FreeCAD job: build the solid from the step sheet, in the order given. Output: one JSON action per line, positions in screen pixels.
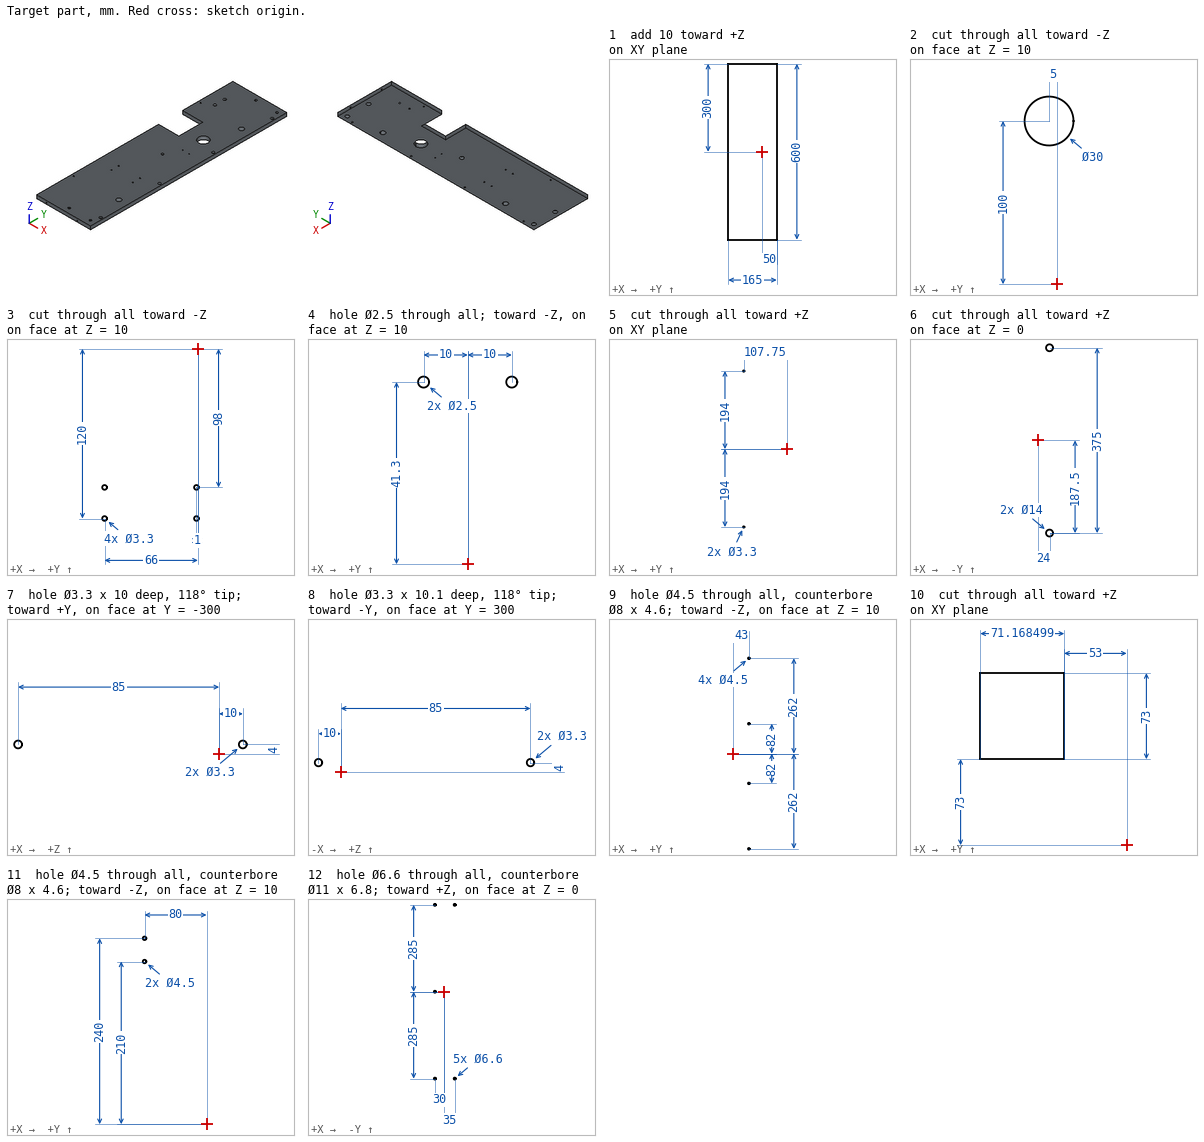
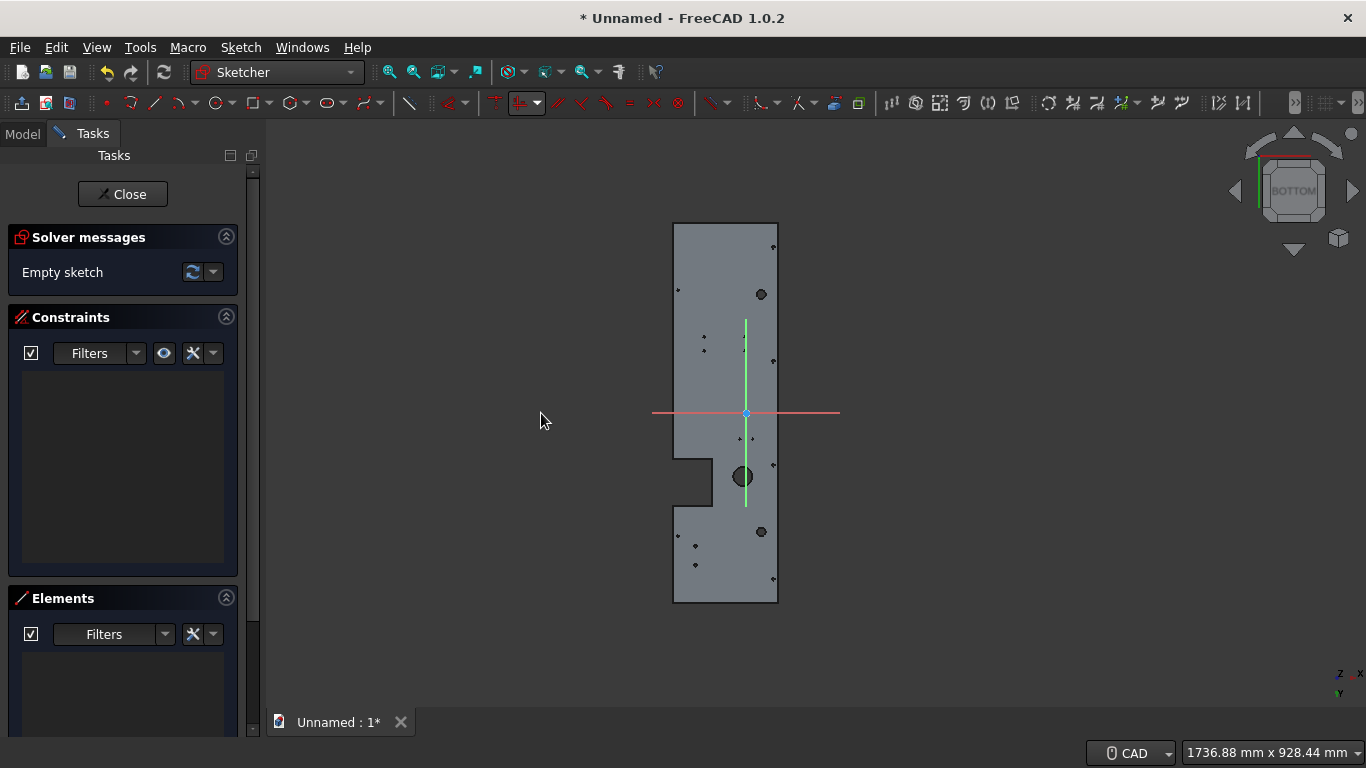
{"action": "left_click", "coordinate": [216, 104]}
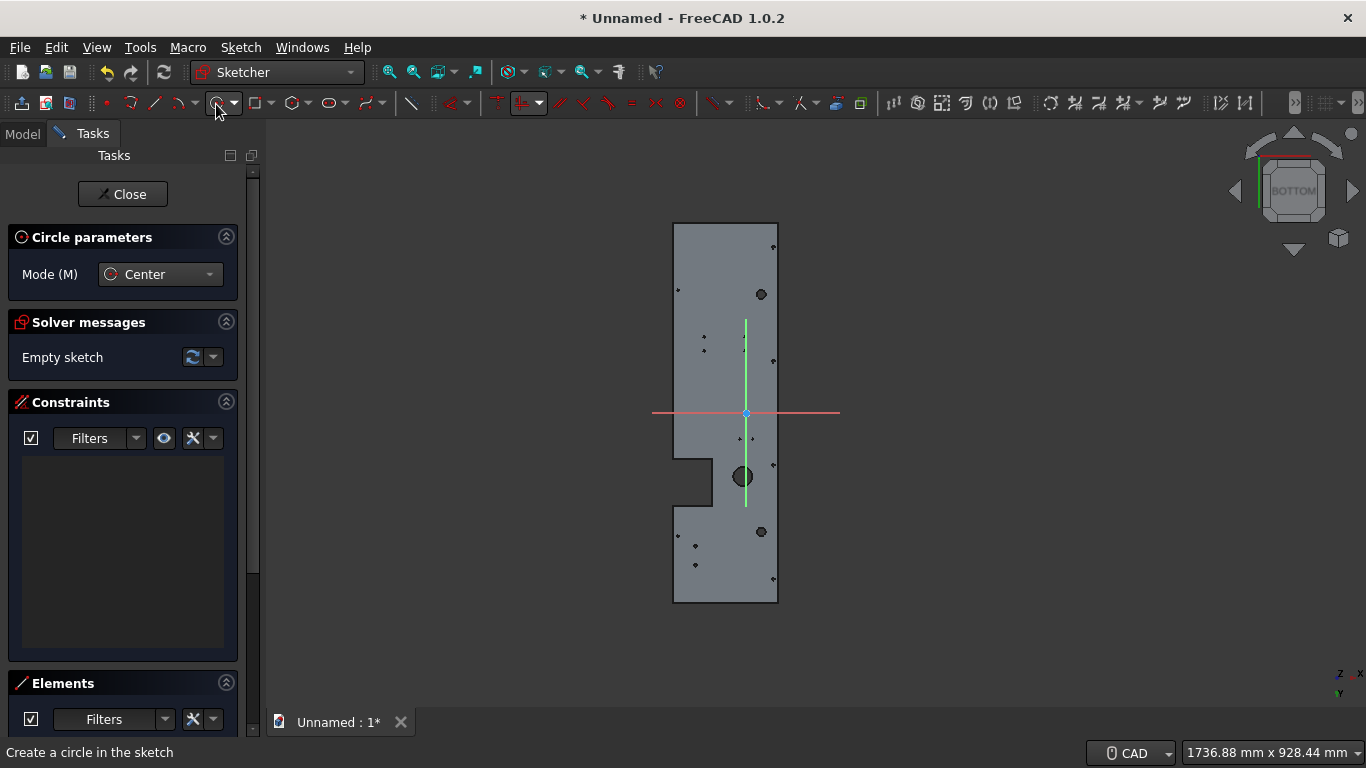
{"action": "scroll", "coordinate": [727, 594], "scroll_direction": "up", "scroll_amount": 12}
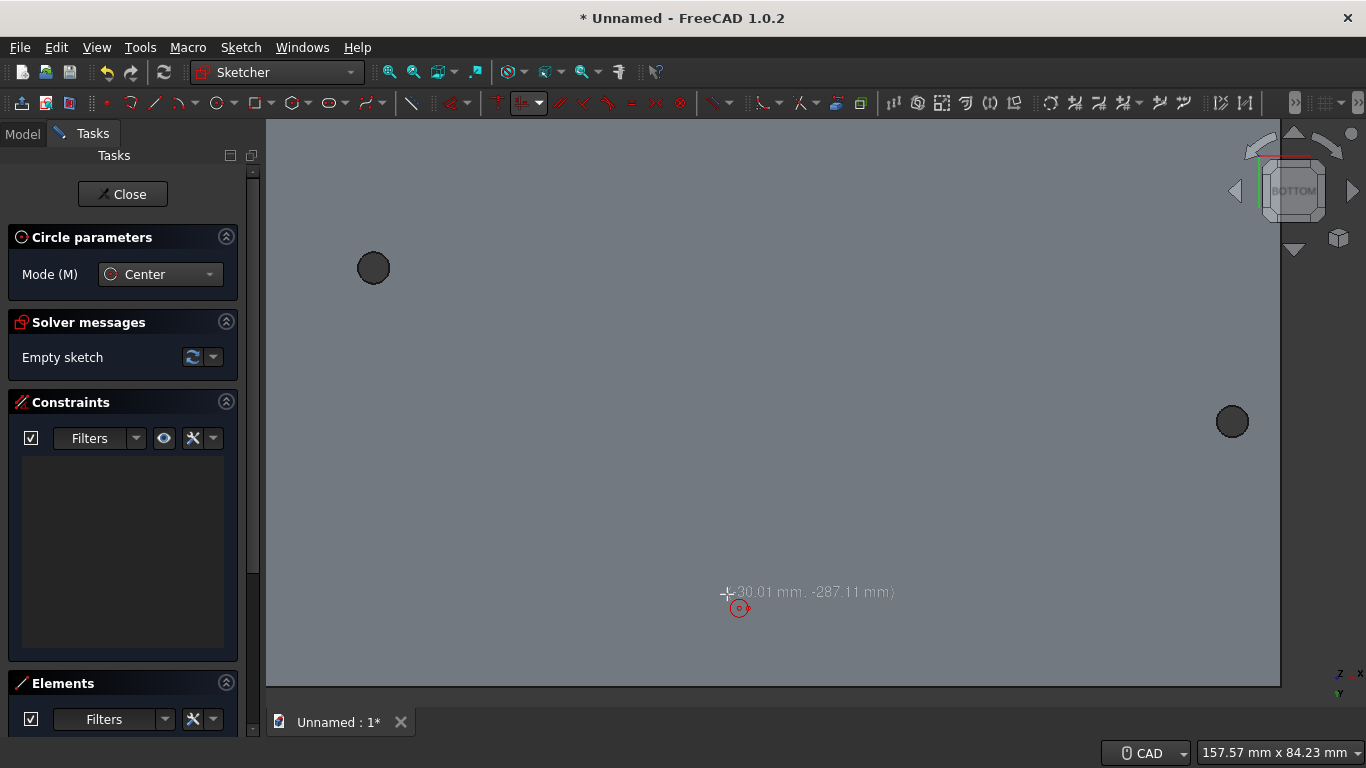
{"action": "scroll", "coordinate": [727, 595], "scroll_direction": "down", "scroll_amount": 12}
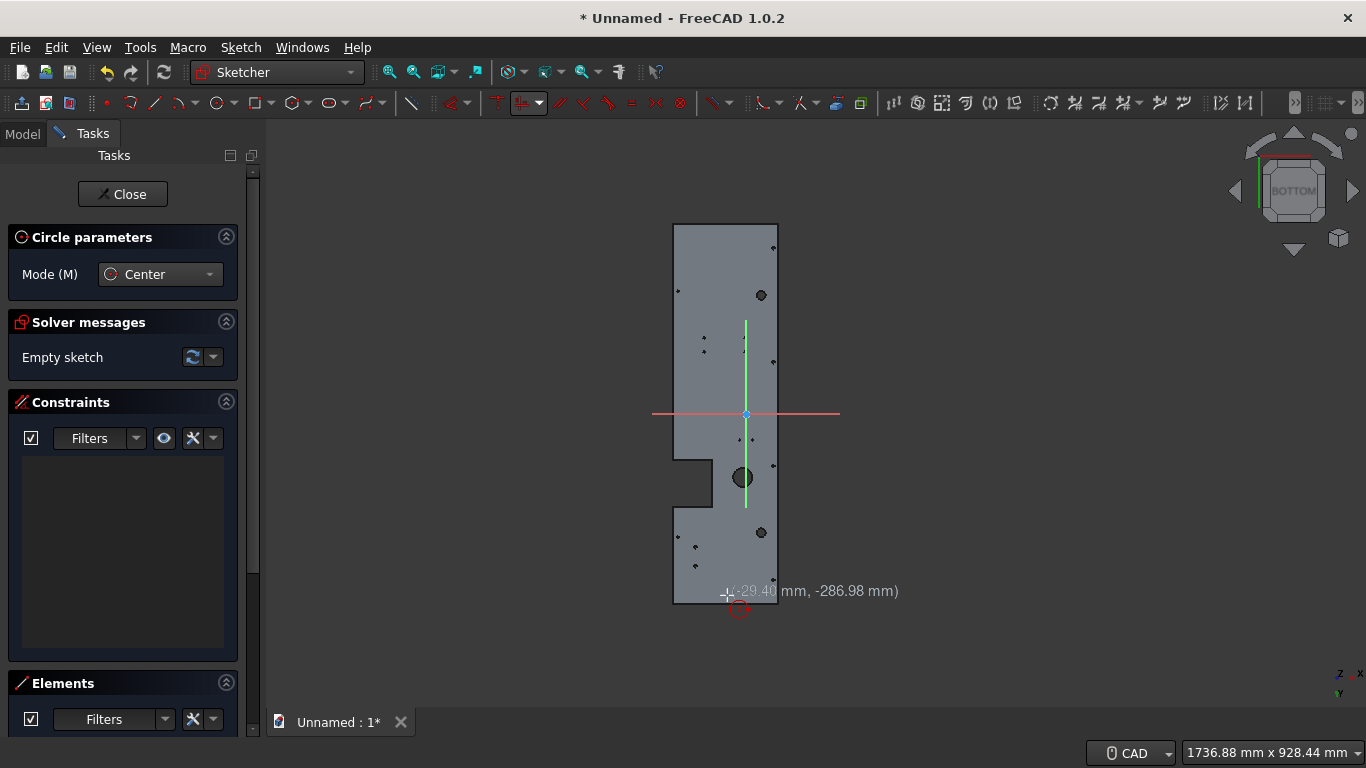
{"action": "left_click", "coordinate": [727, 595]}
{"action": "mouse_move", "coordinate": [728, 593]}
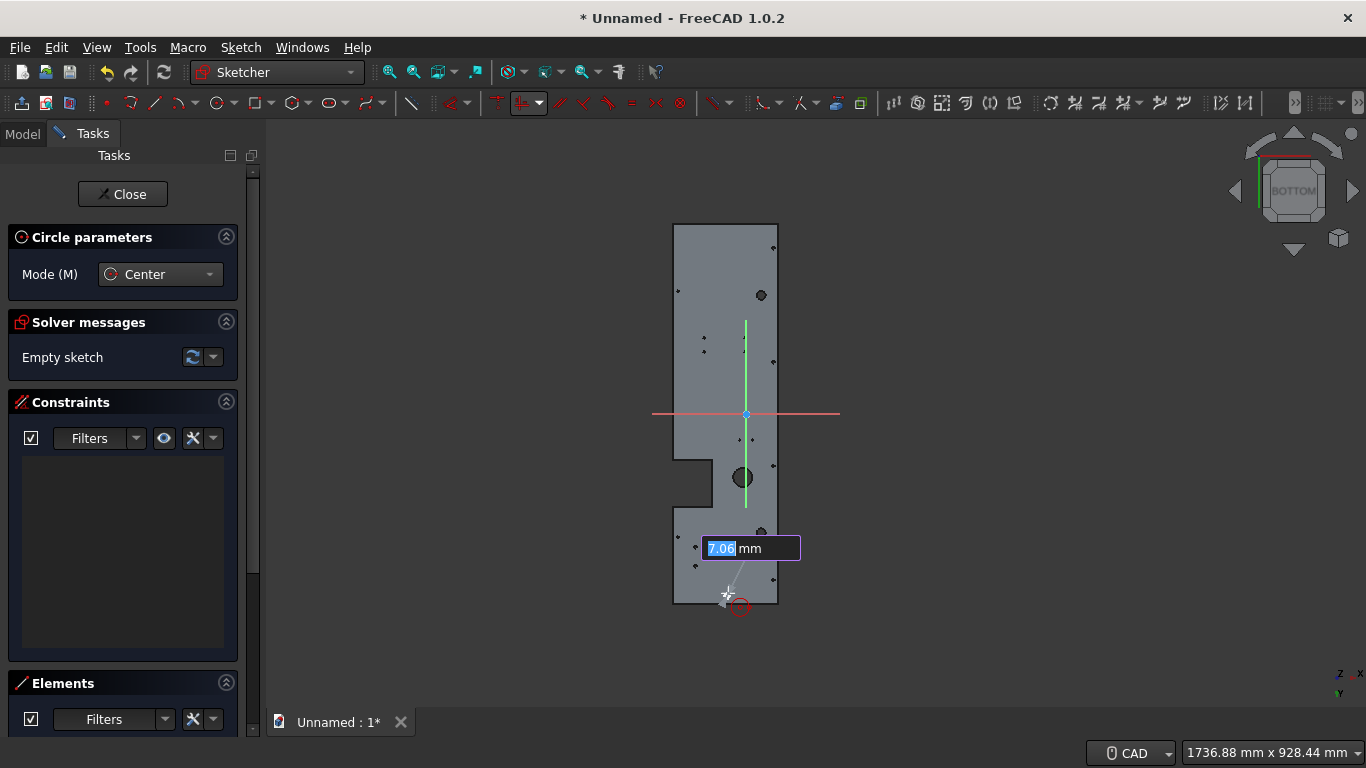
{"action": "type", "text": "6.6"}
{"action": "key", "text": "Return"}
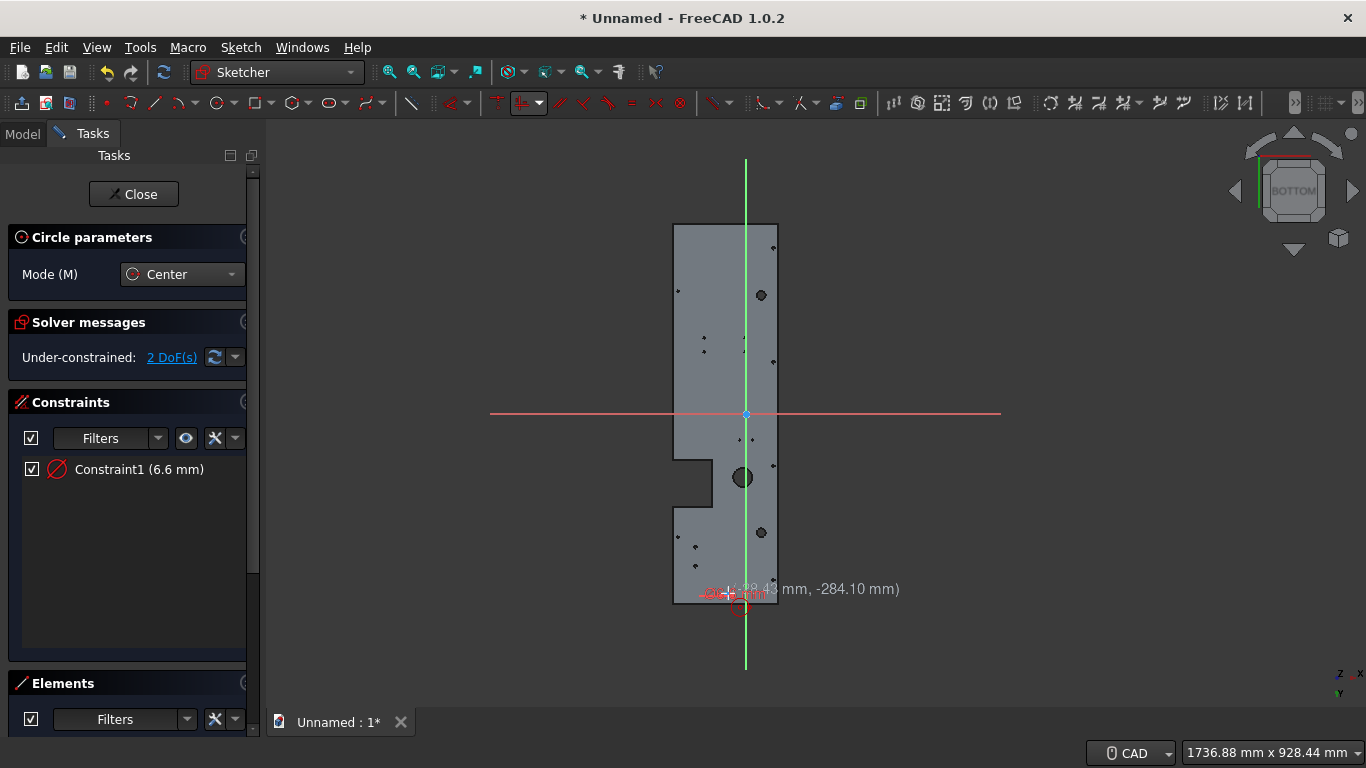
{"action": "scroll", "coordinate": [768, 595], "scroll_direction": "up", "scroll_amount": 12}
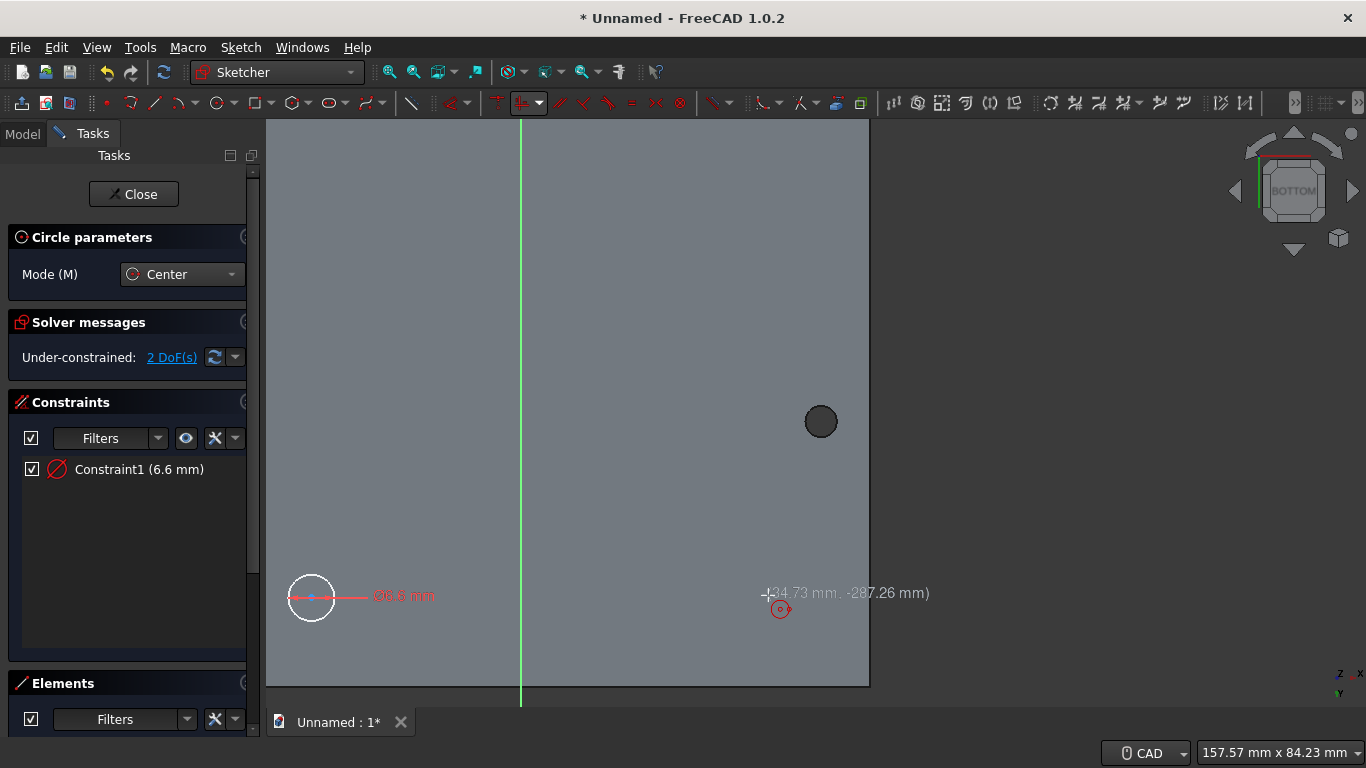
{"action": "scroll", "coordinate": [768, 595], "scroll_direction": "down", "scroll_amount": 12}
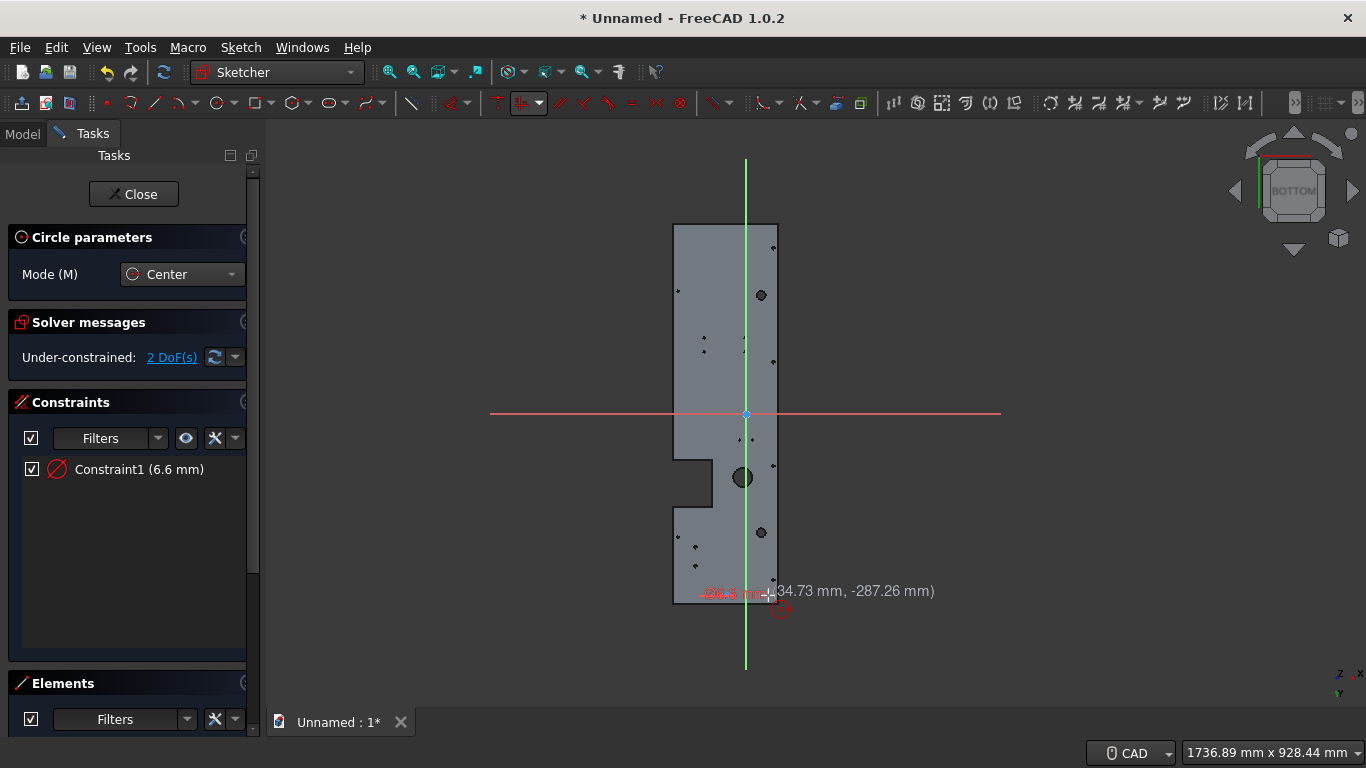
{"action": "left_click", "coordinate": [768, 595]}
{"action": "mouse_move", "coordinate": [770, 593]}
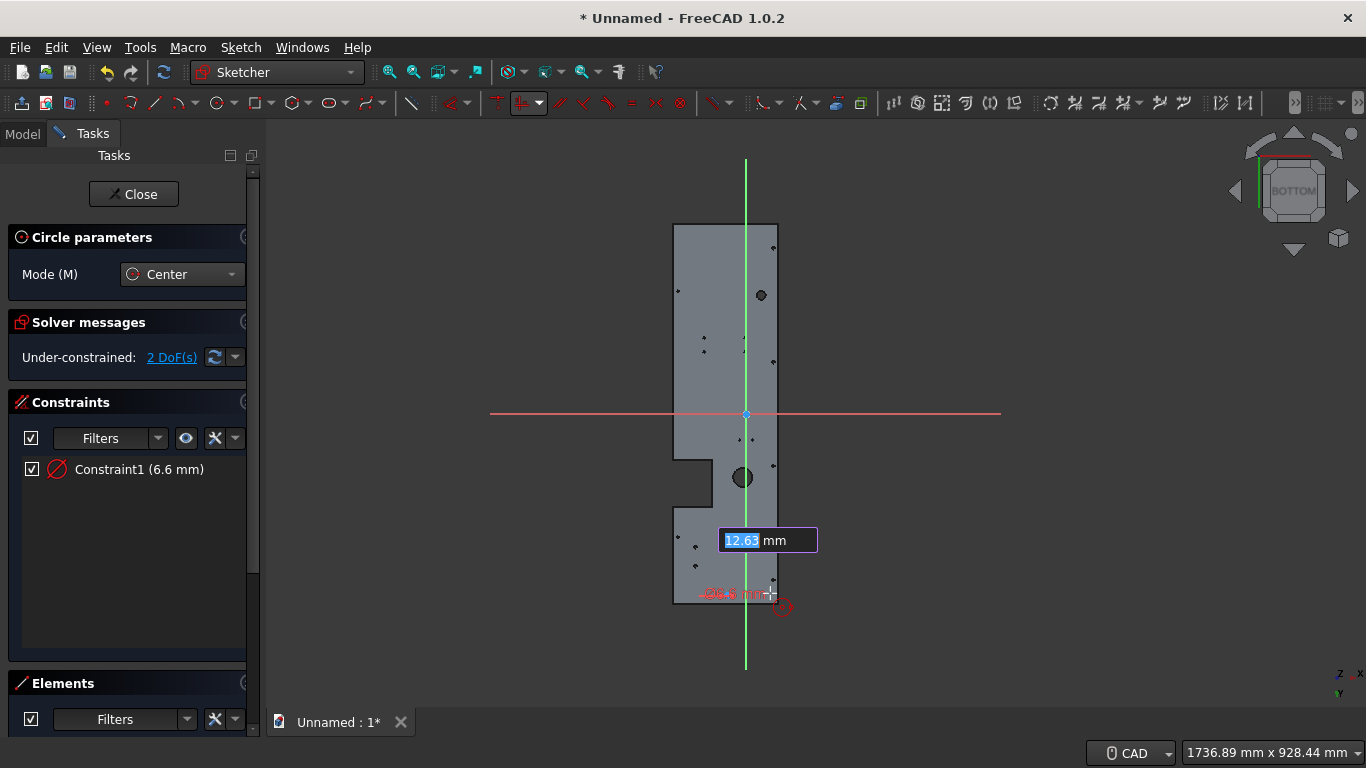
{"action": "type", "text": "6.6"}
{"action": "key", "text": "Return"}